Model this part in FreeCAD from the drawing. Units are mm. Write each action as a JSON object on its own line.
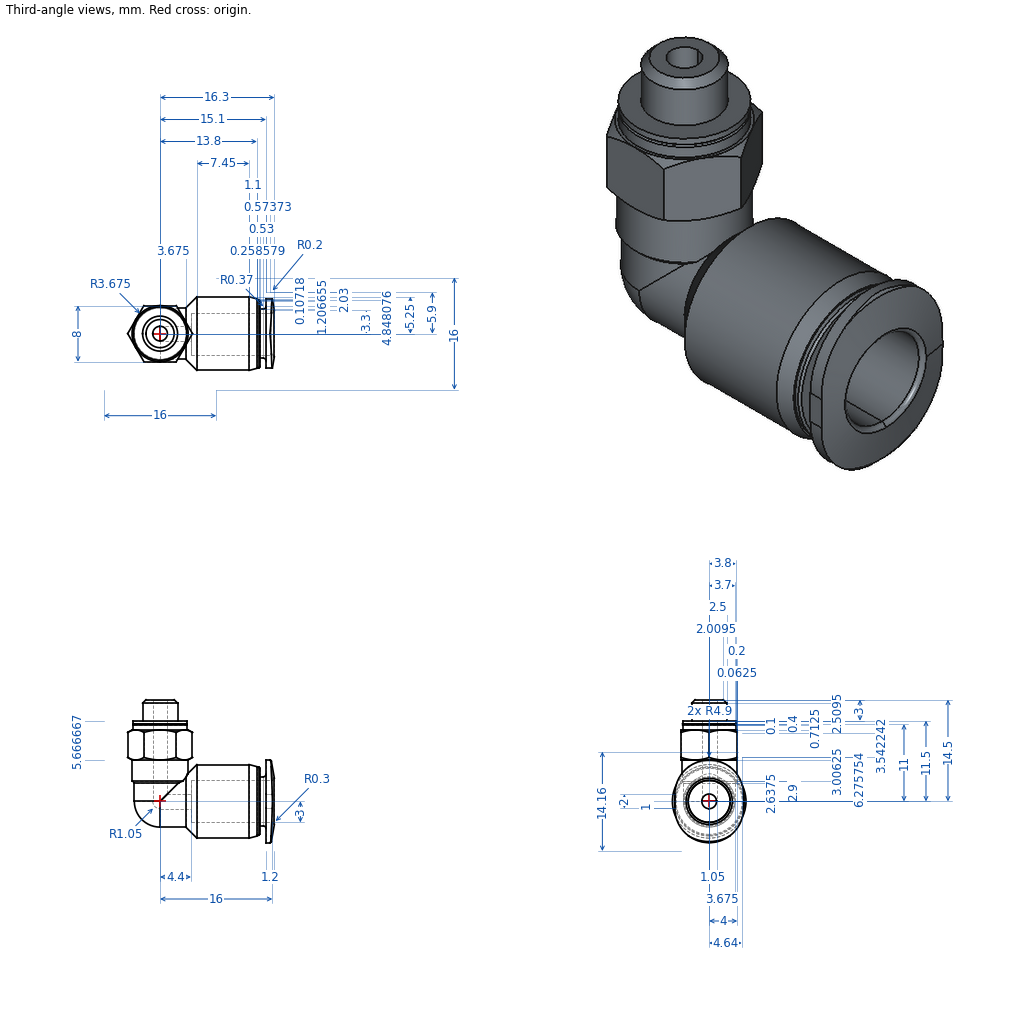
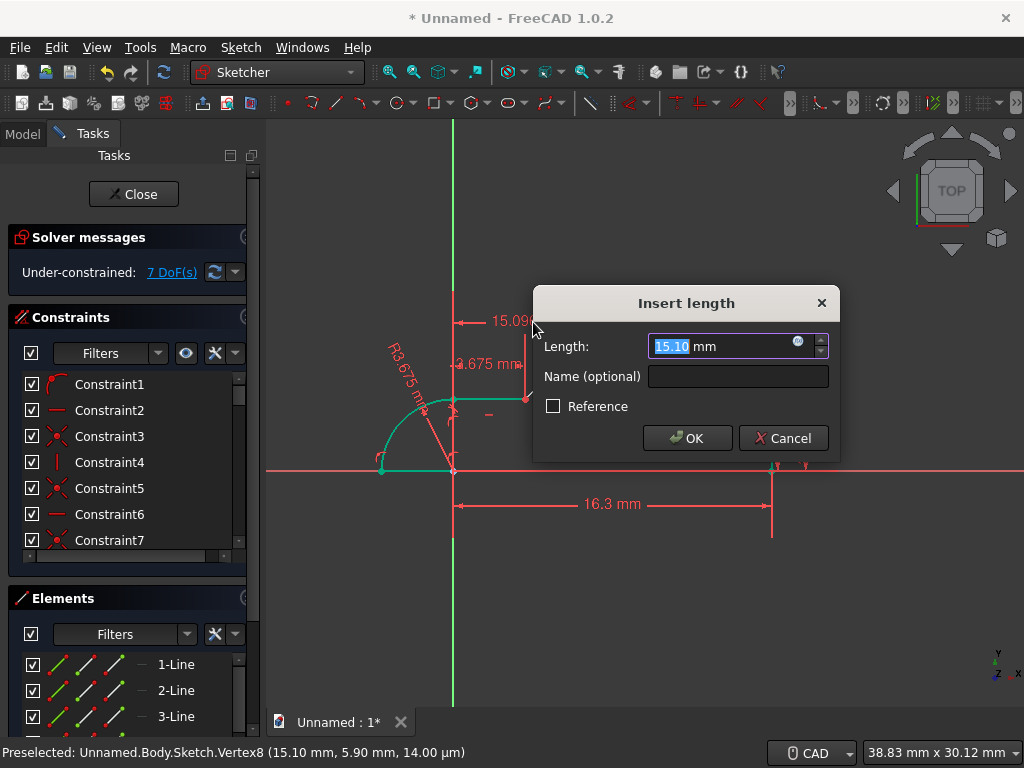
{"action": "type", "text": "15.1"}
{"action": "key", "text": "Return"}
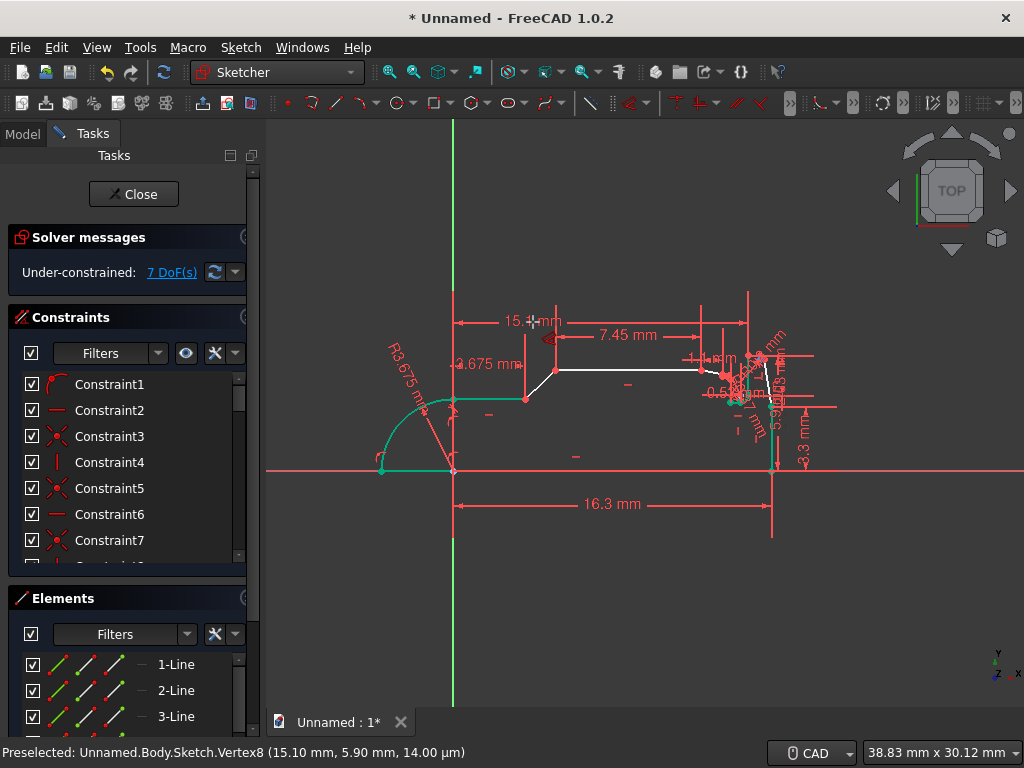
{"action": "scroll", "coordinate": [723, 377], "scroll_direction": "up", "scroll_amount": 9}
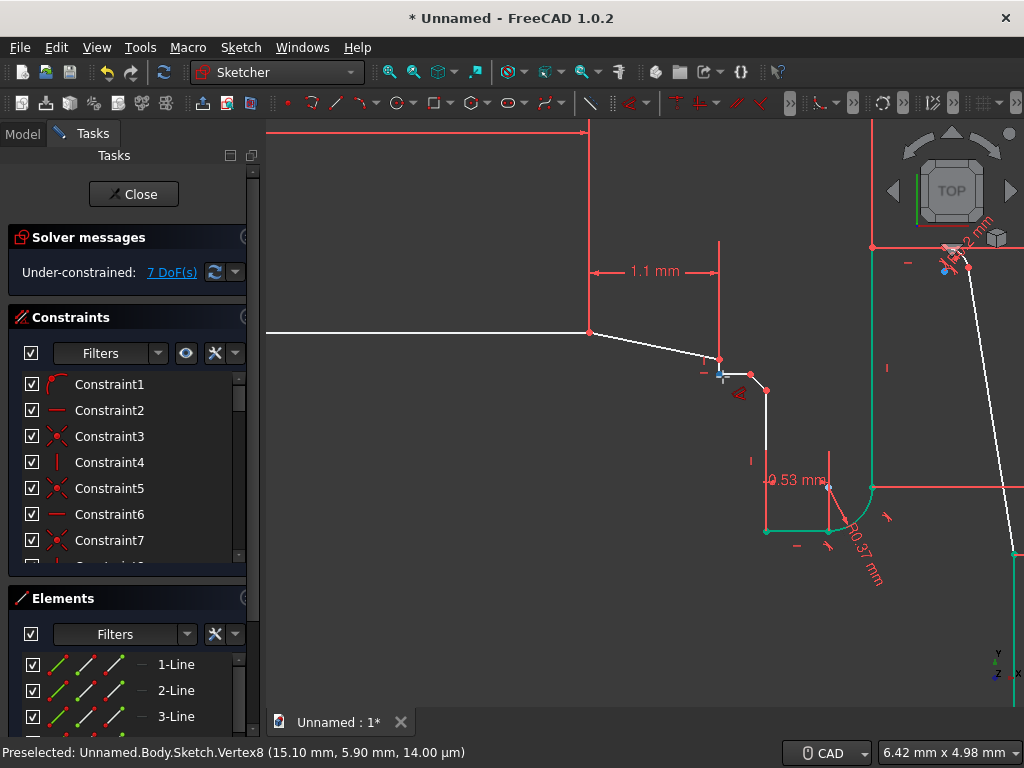
{"action": "left_click", "coordinate": [719, 374]}
{"action": "left_click", "coordinate": [507, 316]}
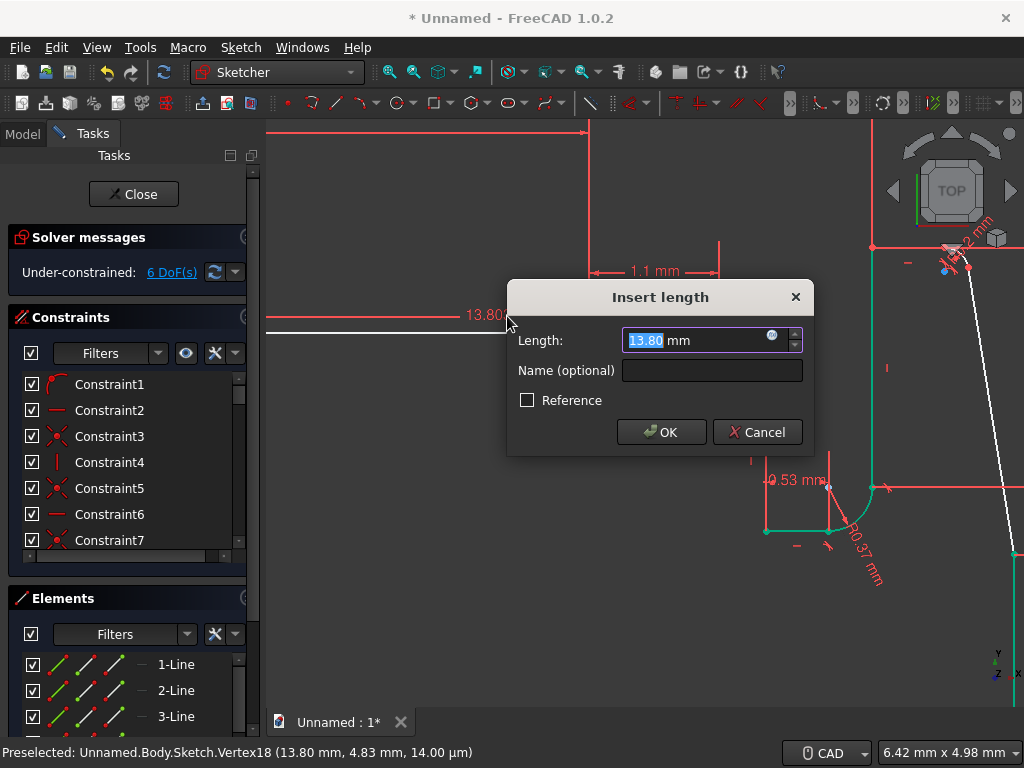
{"action": "type", "text": "13.8"}
{"action": "key", "text": "Return"}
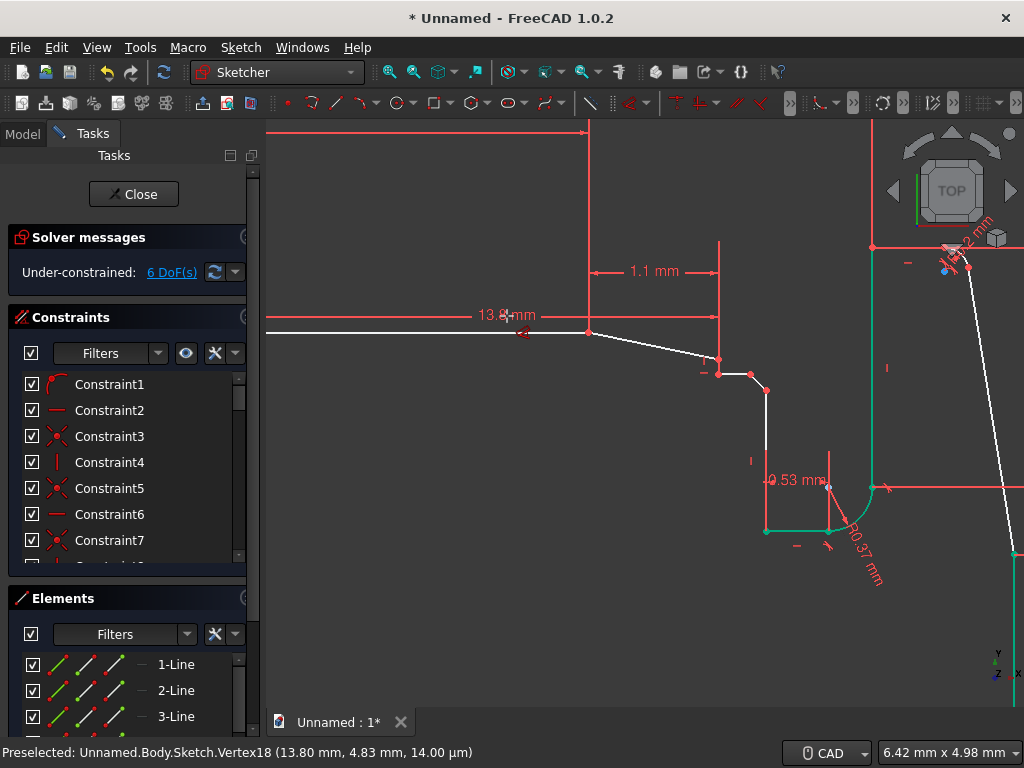
{"action": "scroll", "coordinate": [723, 377], "scroll_direction": "down", "scroll_amount": 9}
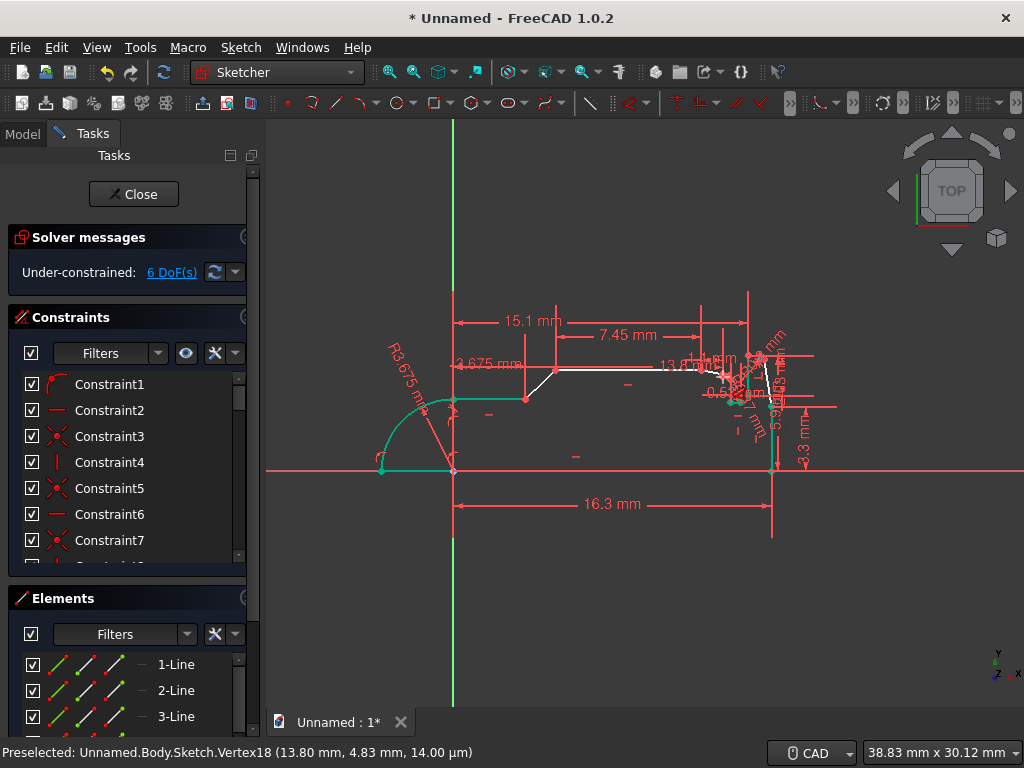
{"action": "left_click", "coordinate": [701, 370]}
{"action": "left_click", "coordinate": [419, 444]}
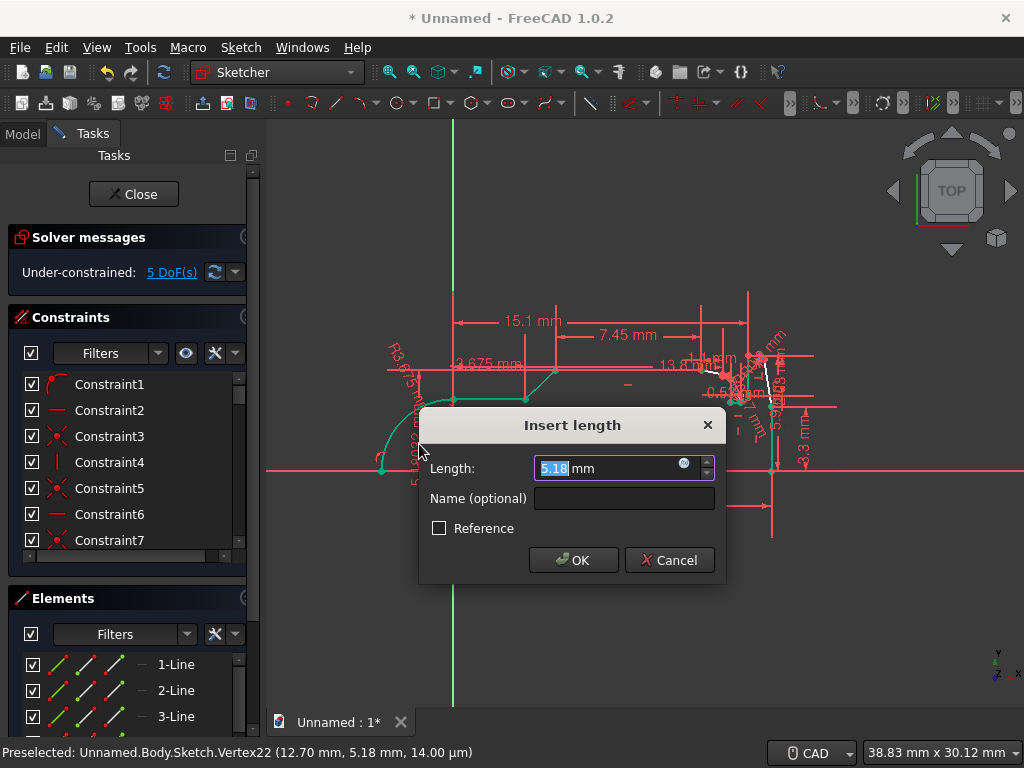
{"action": "type", "text": "5.25"}
{"action": "key", "text": "Return"}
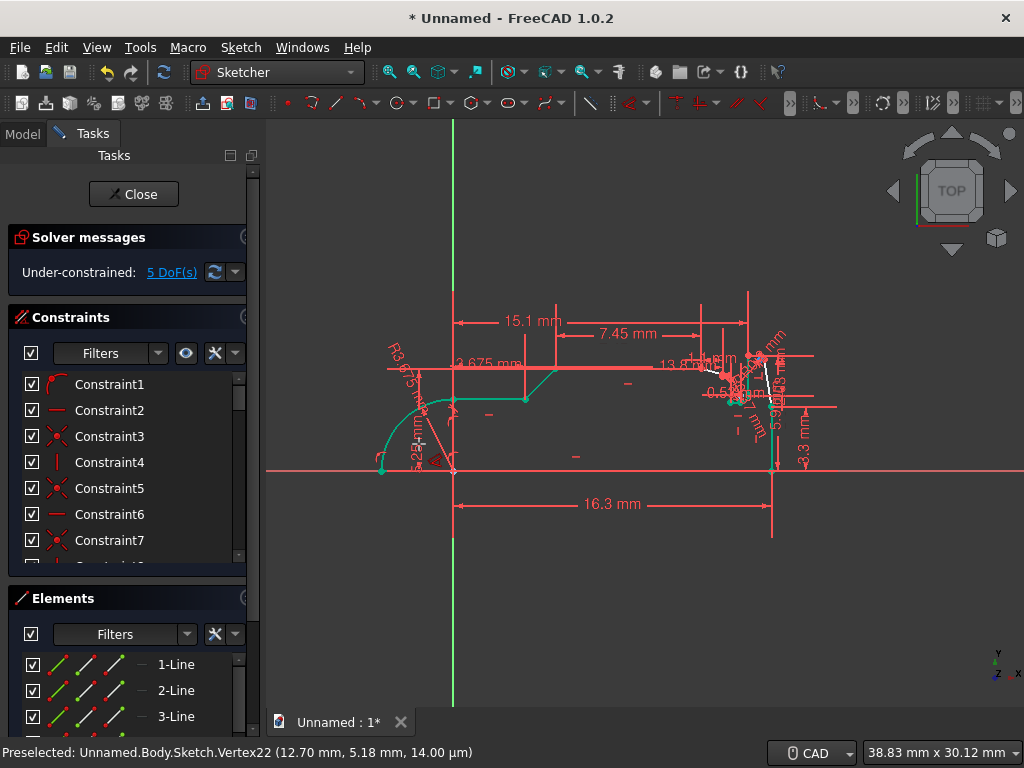
{"action": "scroll", "coordinate": [754, 356], "scroll_direction": "up", "scroll_amount": 7}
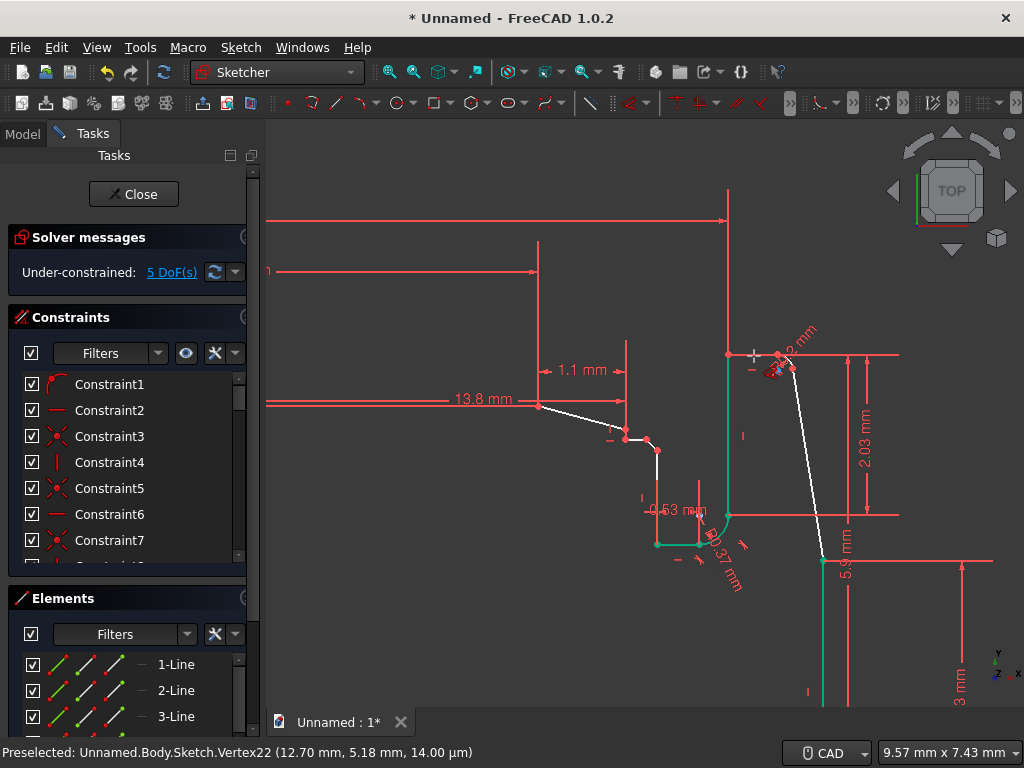
{"action": "left_click", "coordinate": [753, 355]}
{"action": "left_click", "coordinate": [753, 321]}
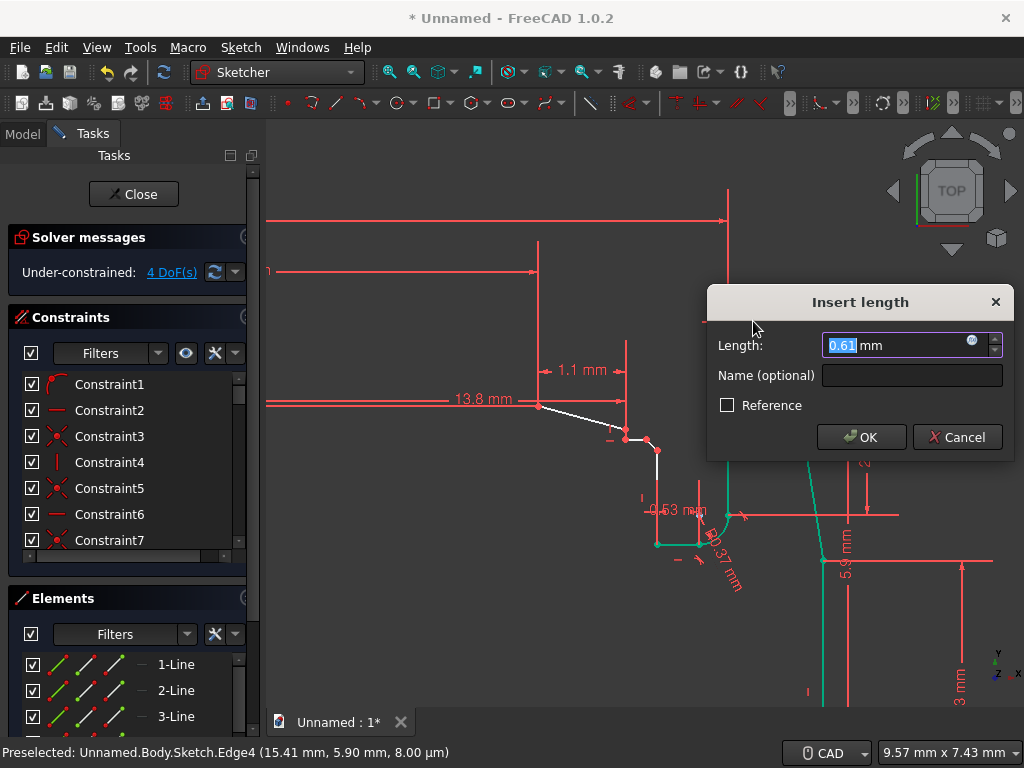
{"action": "type", "text": "0.57373"}
{"action": "key", "text": "Return"}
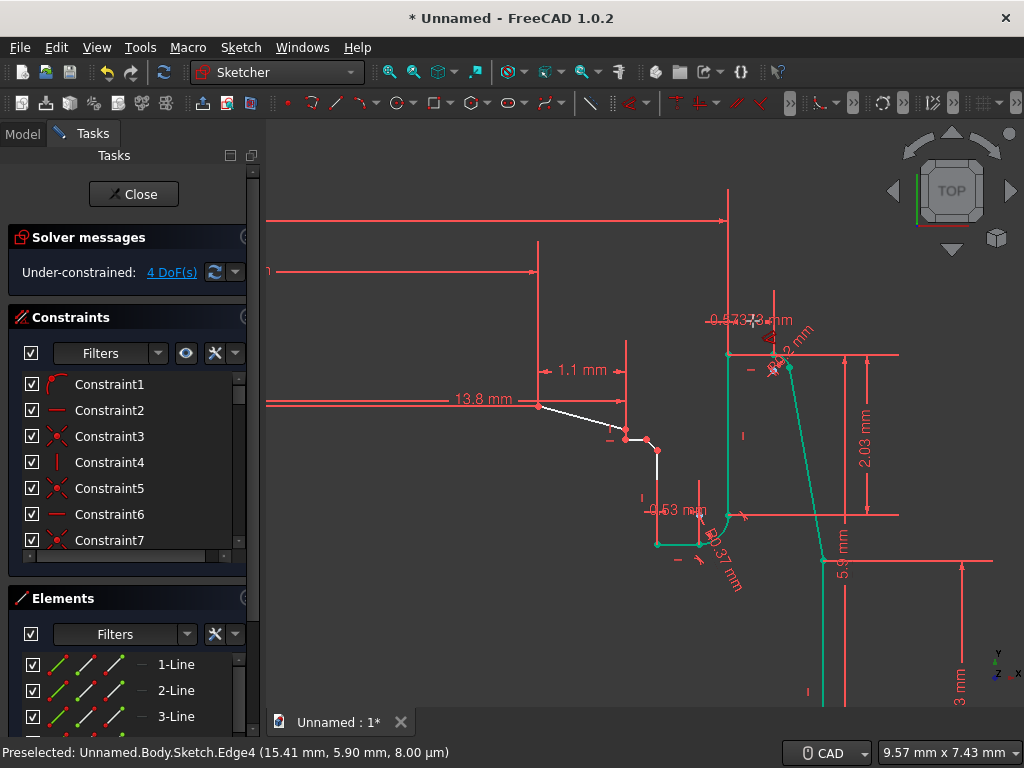
{"action": "scroll", "coordinate": [626, 435], "scroll_direction": "up", "scroll_amount": 8}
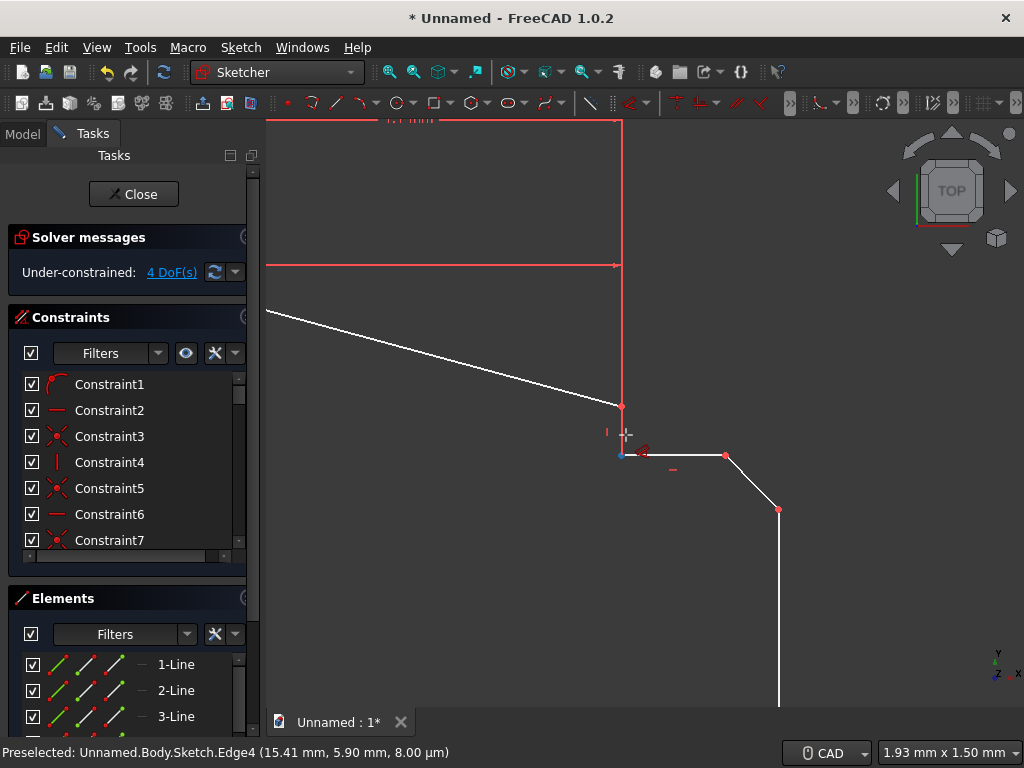
{"action": "left_click", "coordinate": [622, 431]}
{"action": "left_click", "coordinate": [656, 431]}